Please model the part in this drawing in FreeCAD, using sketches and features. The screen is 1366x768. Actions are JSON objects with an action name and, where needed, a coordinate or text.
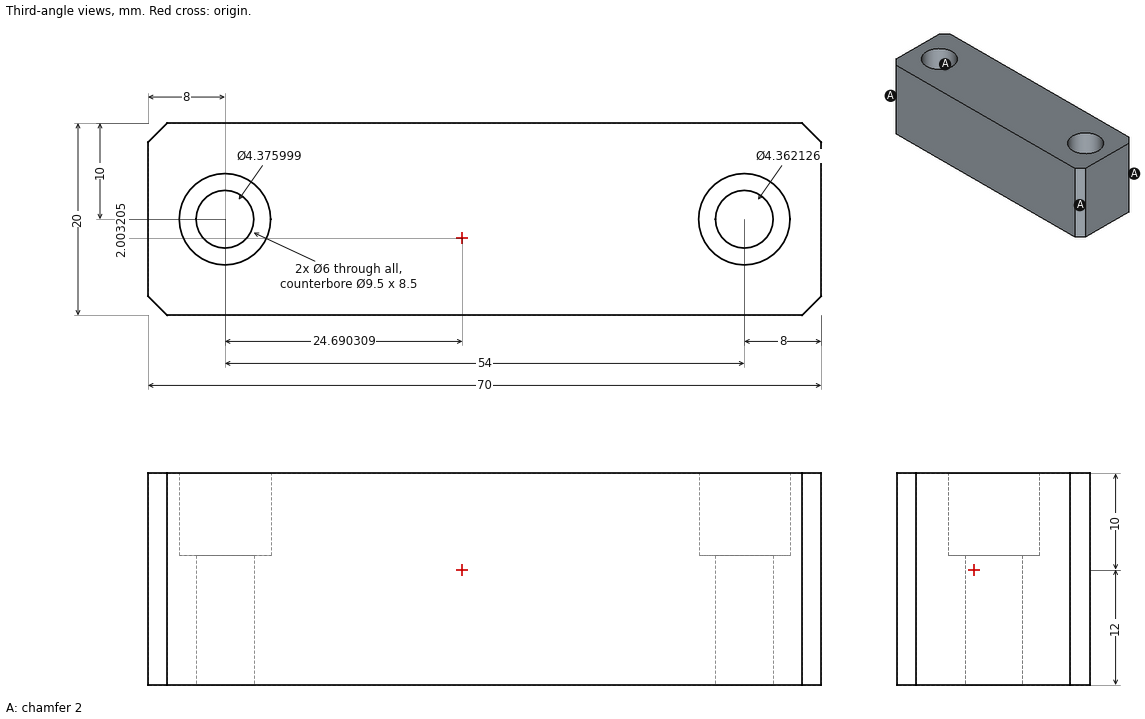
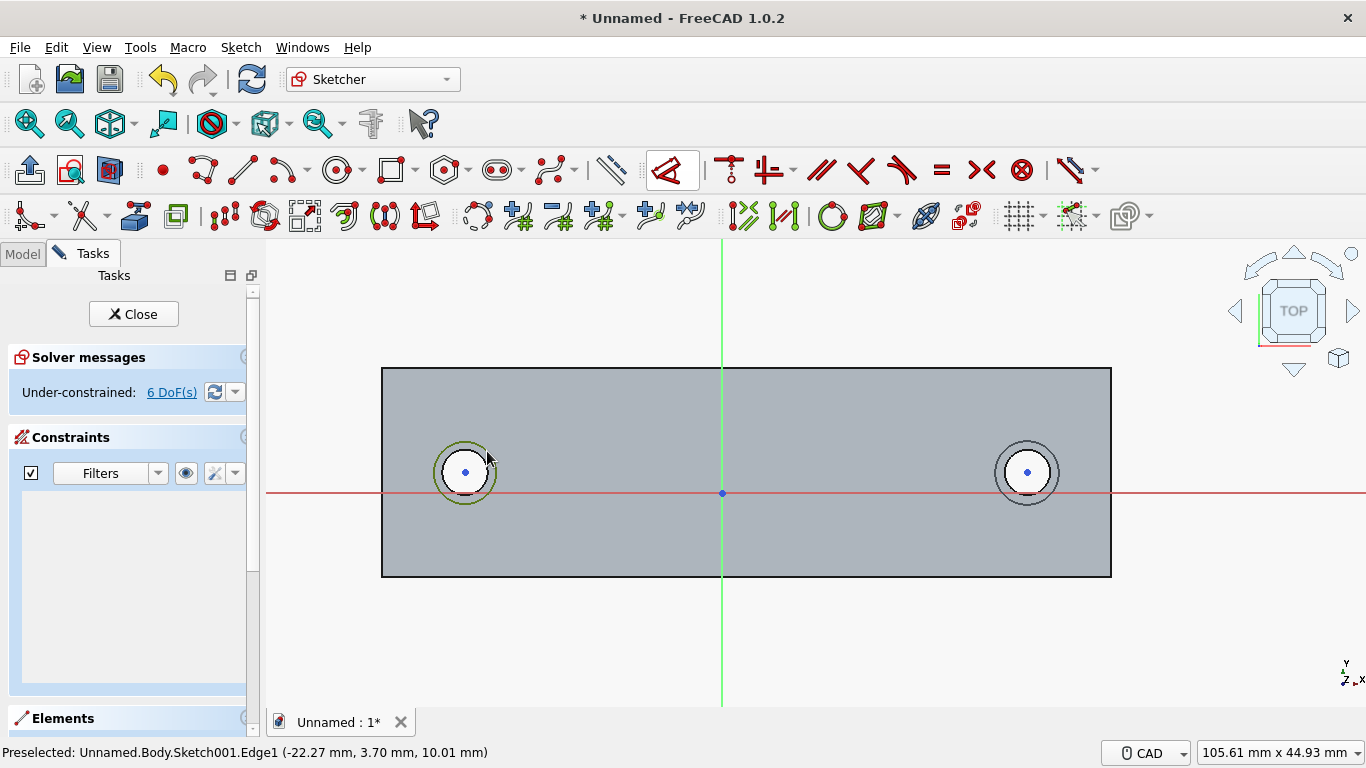
{"action": "left_click", "coordinate": [1049, 450]}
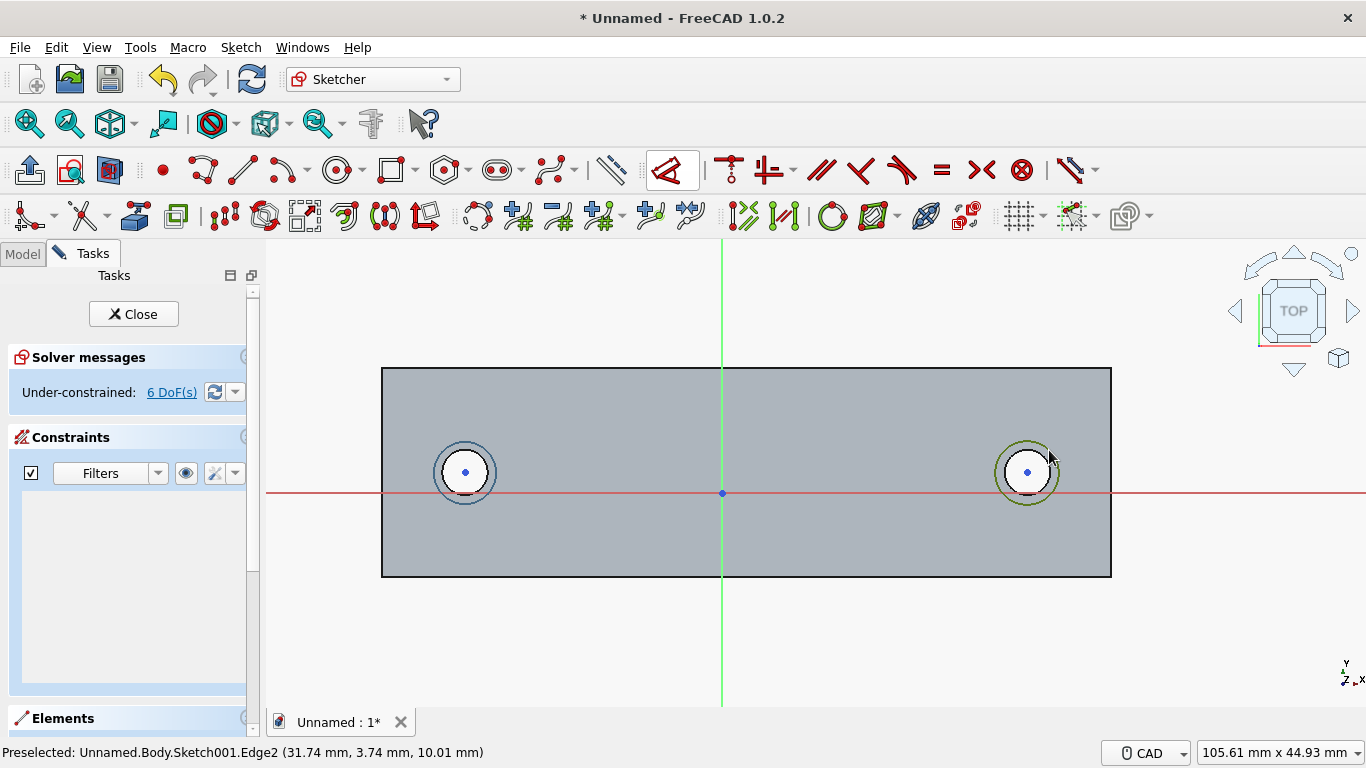
{"action": "key", "text": "e"}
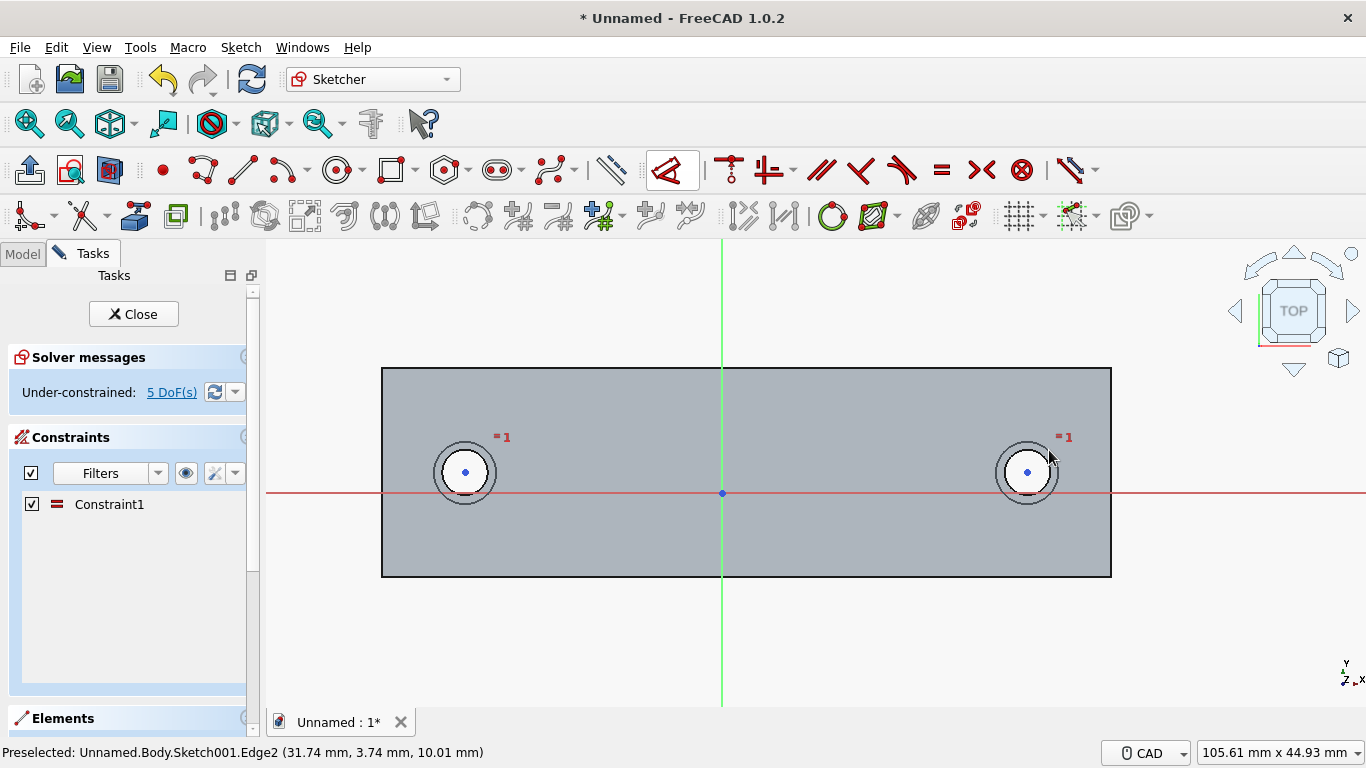
{"action": "left_click", "coordinate": [465, 473]}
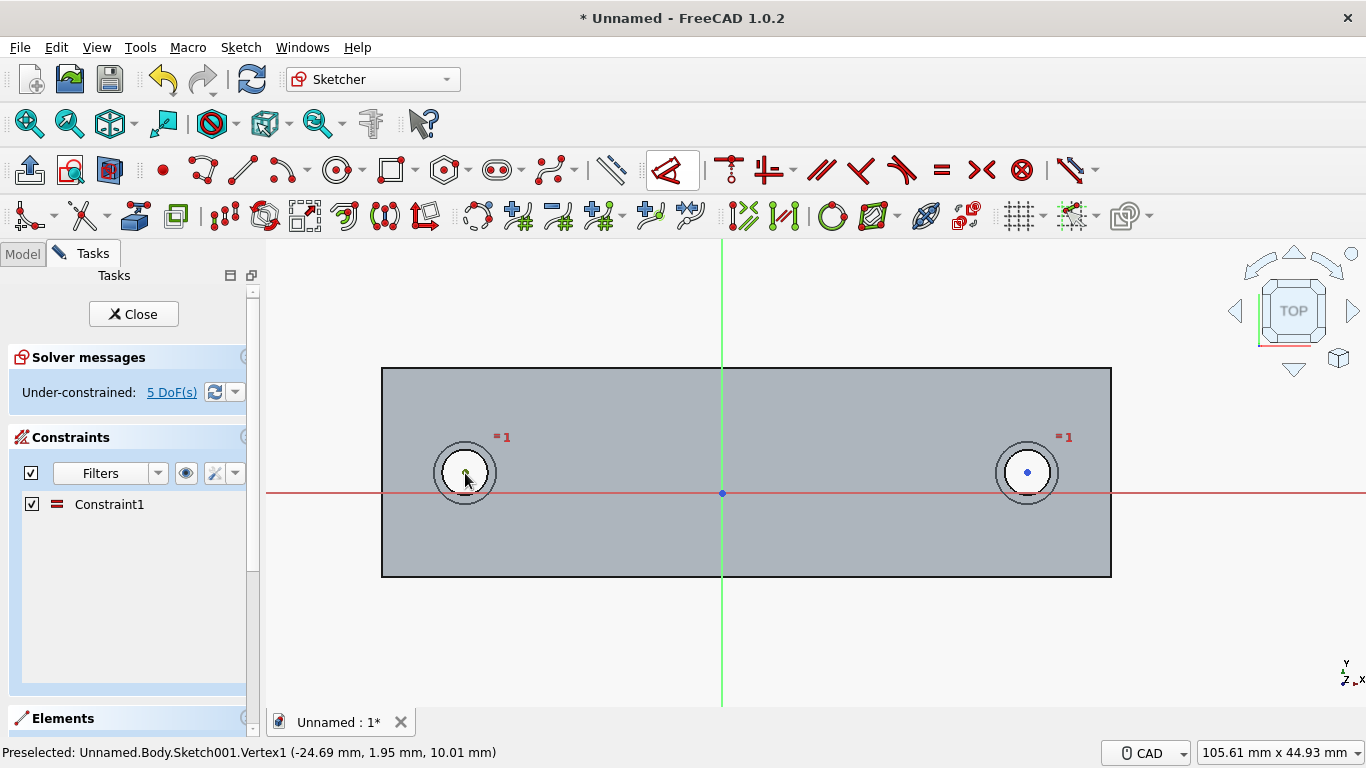
{"action": "left_click", "coordinate": [1027, 473]}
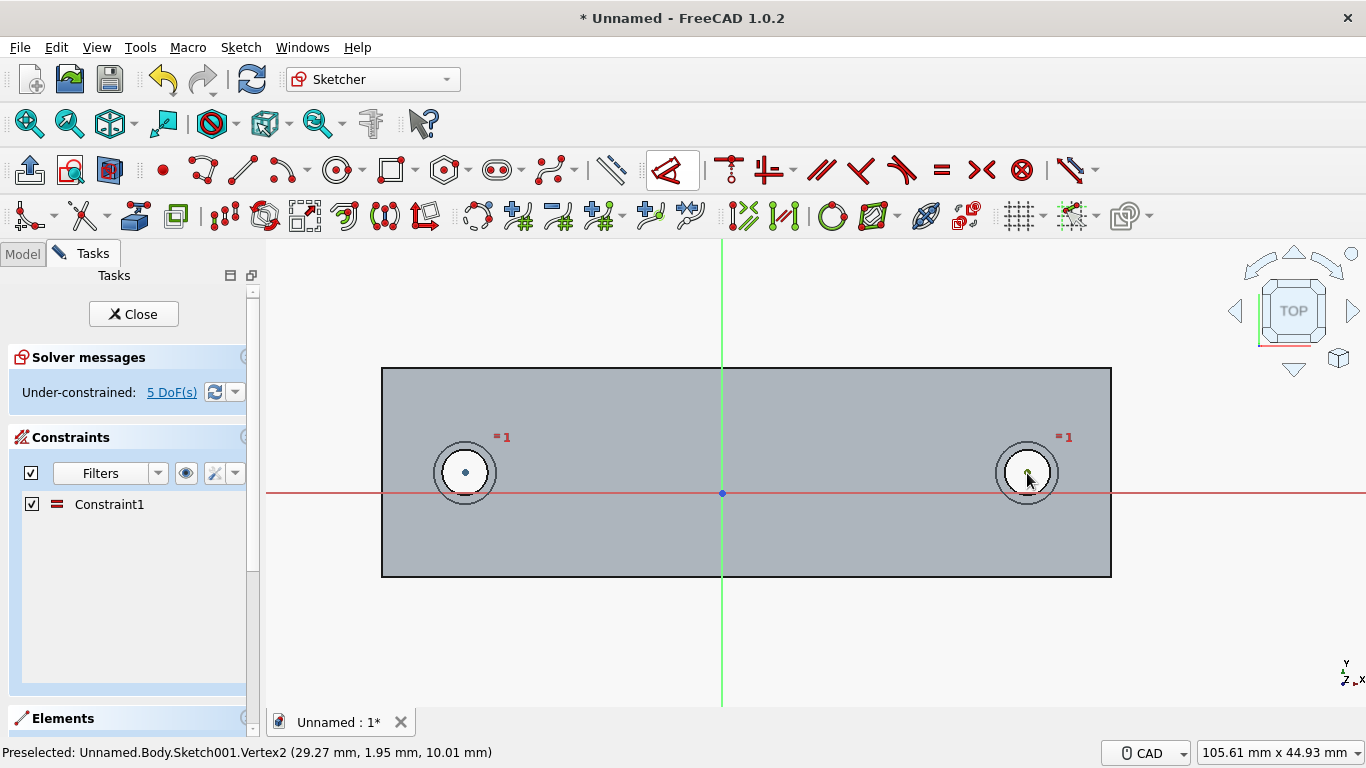
{"action": "key", "text": "h"}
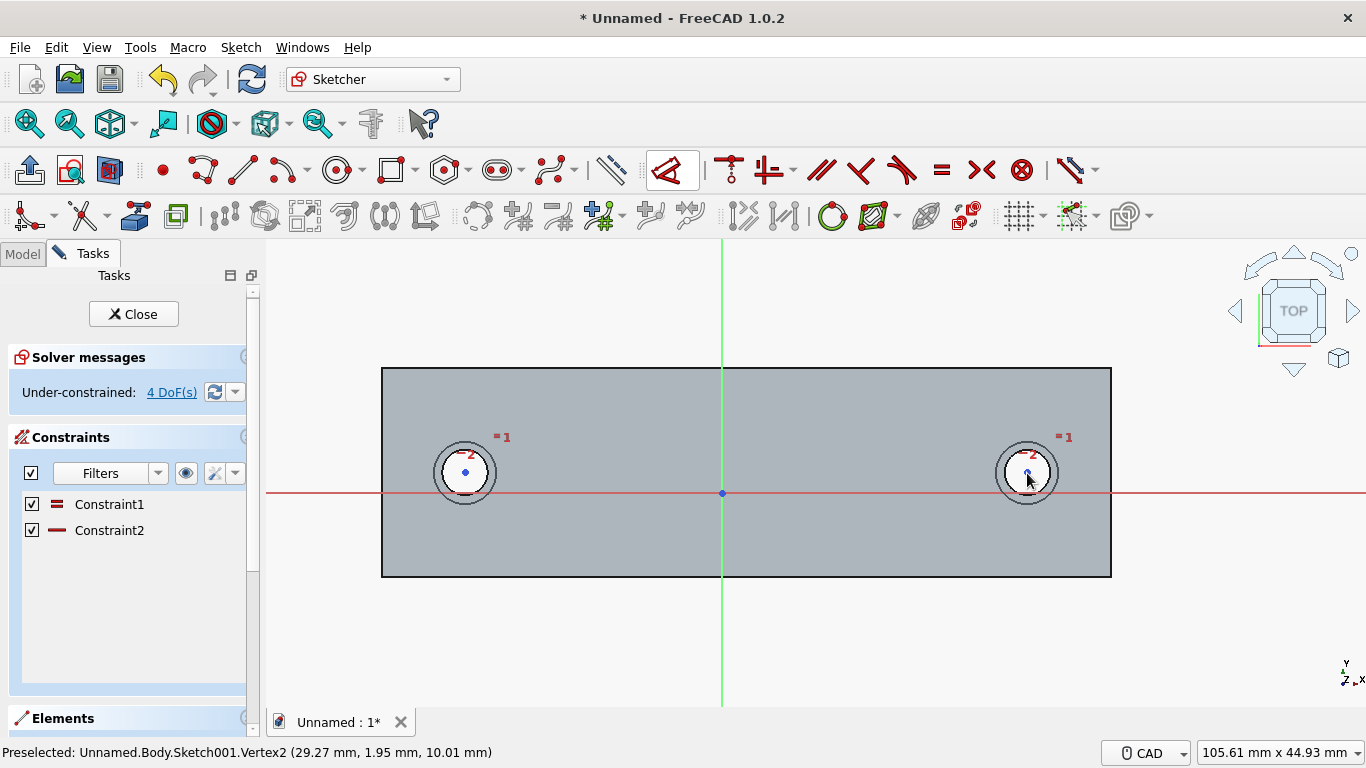
{"action": "left_click", "coordinate": [487, 451]}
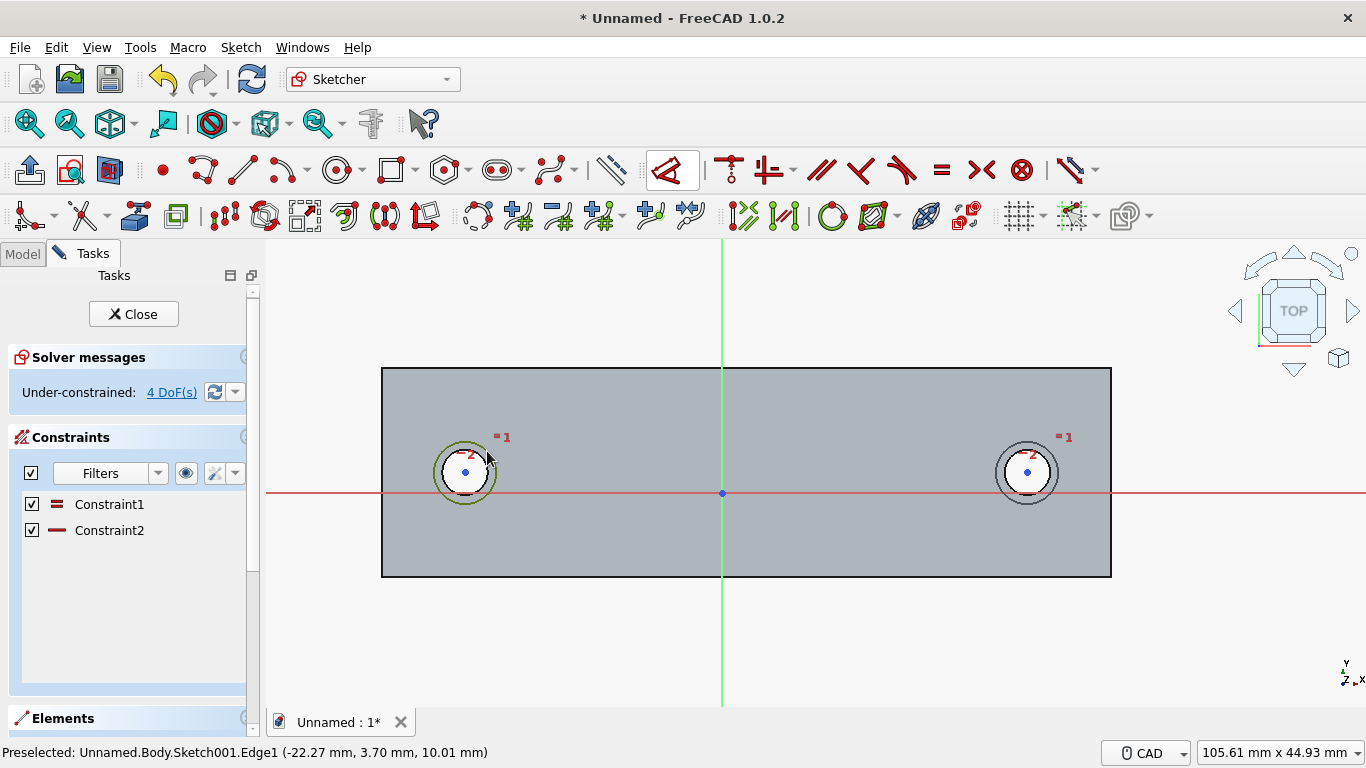
{"action": "left_click", "coordinate": [694, 170]}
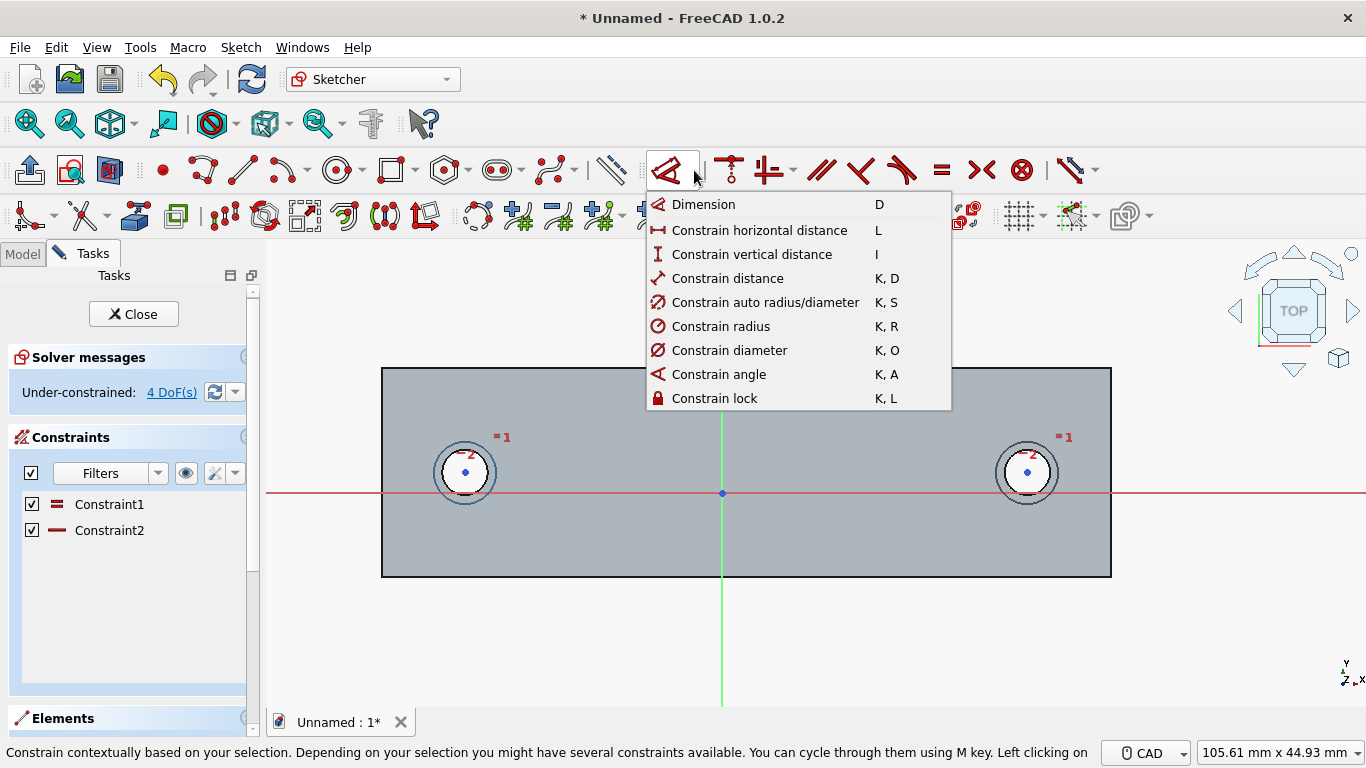
{"action": "left_click", "coordinate": [799, 350]}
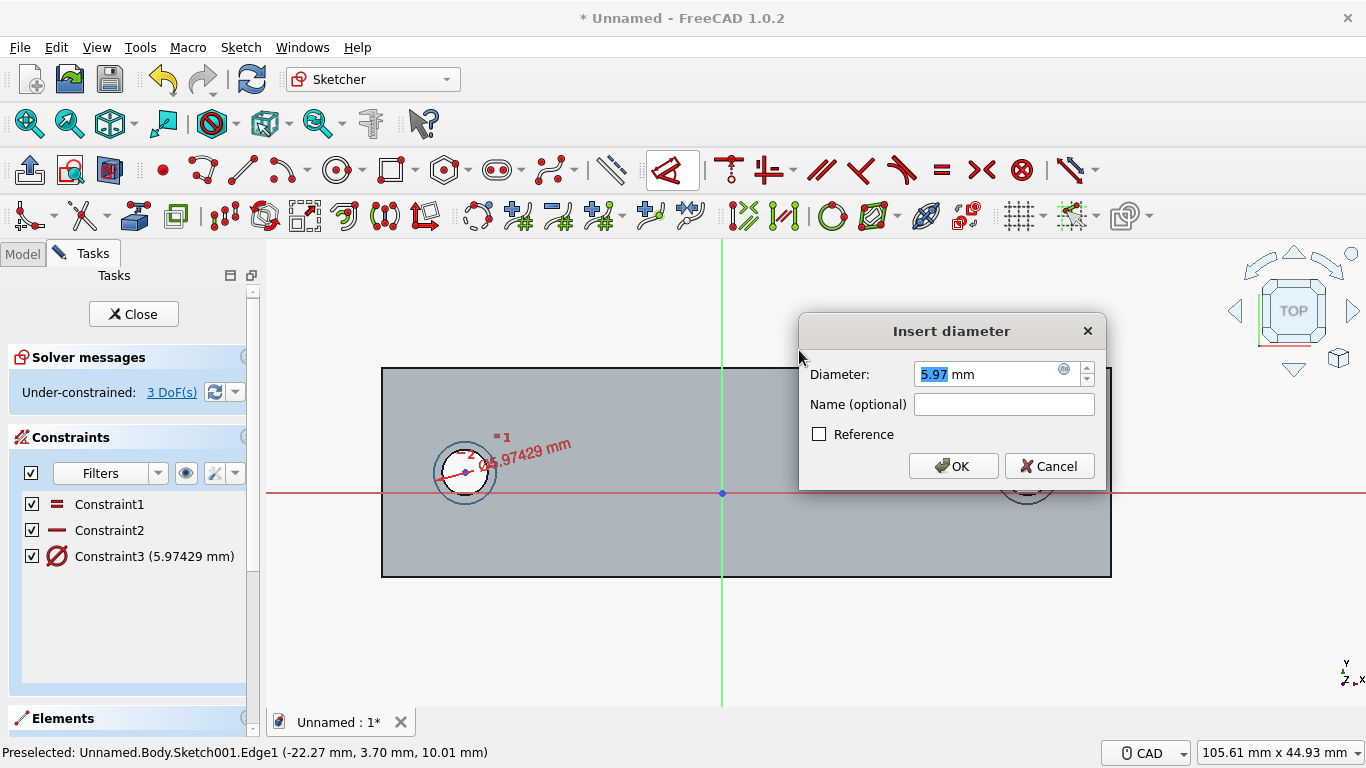
{"action": "type", "text": "6"}
{"action": "key", "text": "Return"}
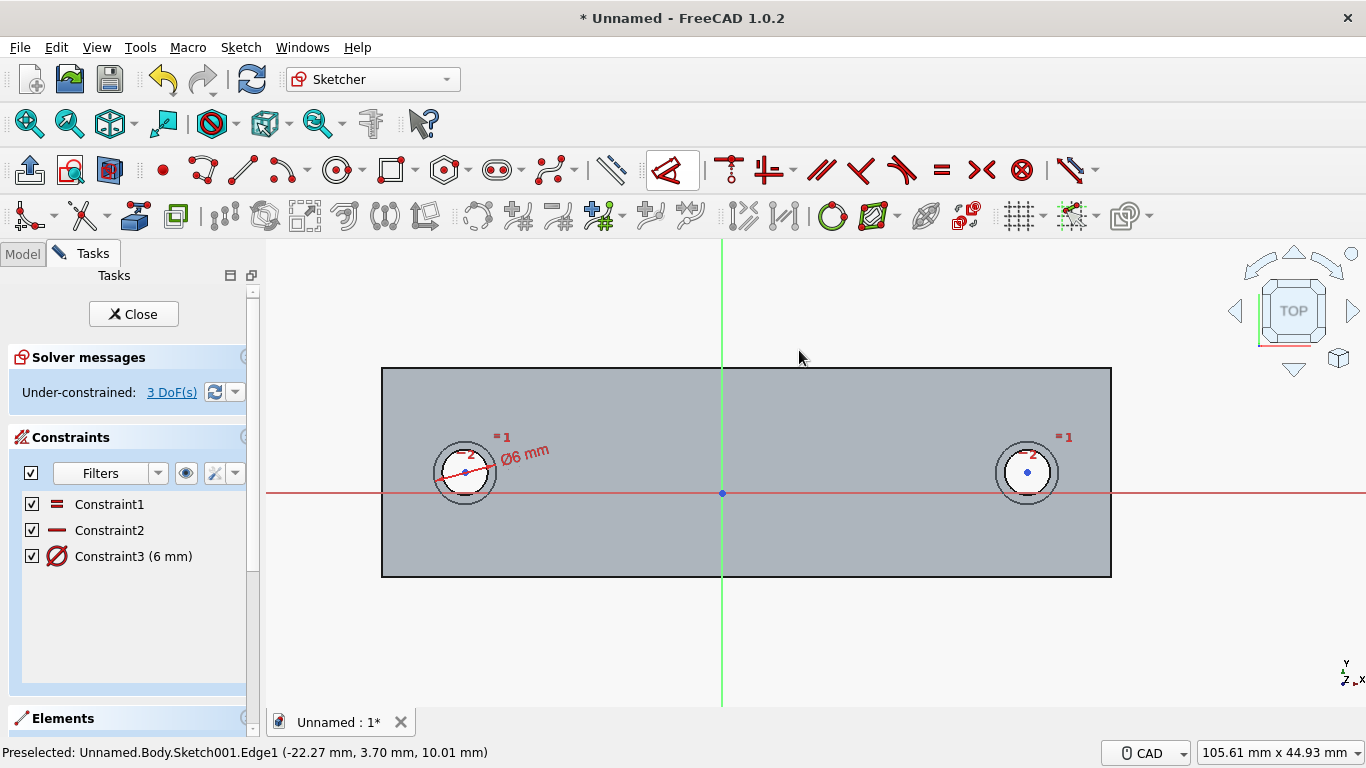
{"action": "left_click", "coordinate": [465, 473]}